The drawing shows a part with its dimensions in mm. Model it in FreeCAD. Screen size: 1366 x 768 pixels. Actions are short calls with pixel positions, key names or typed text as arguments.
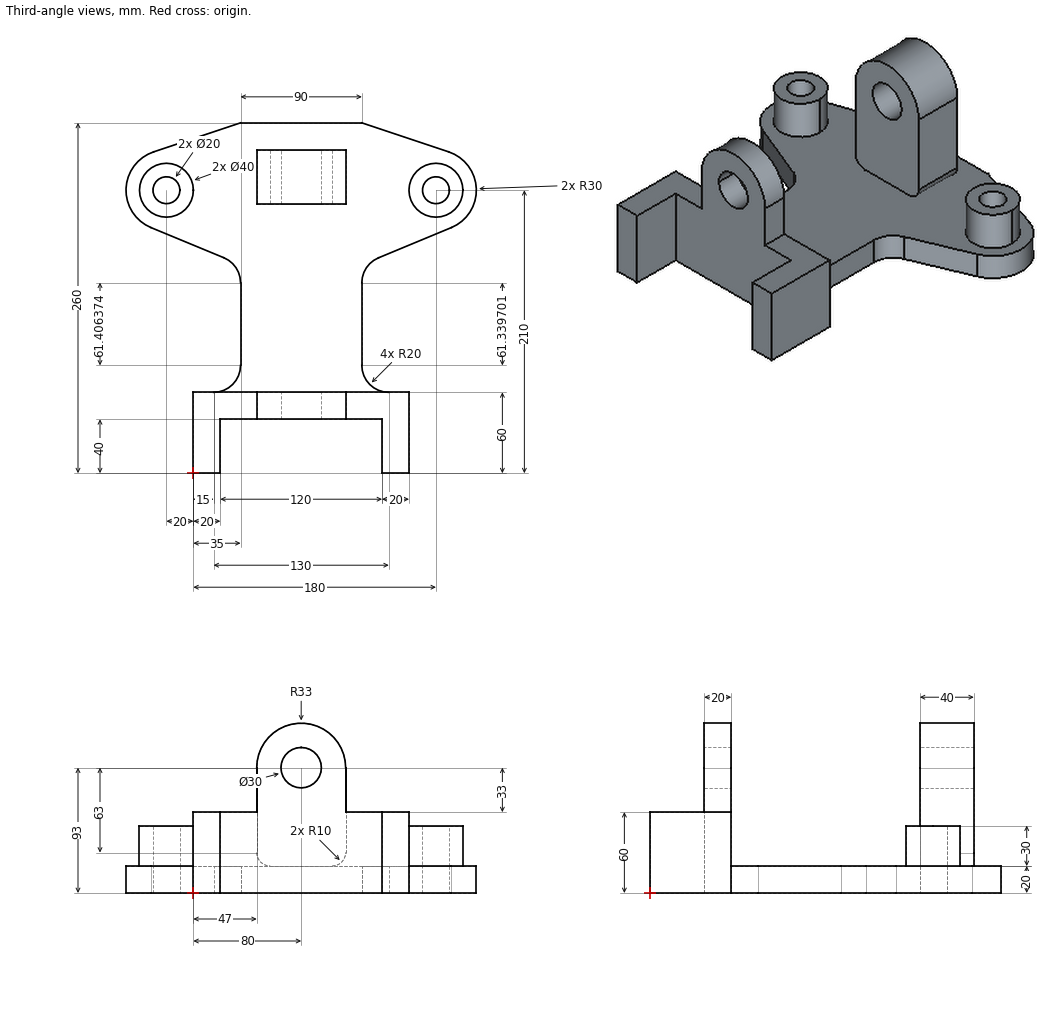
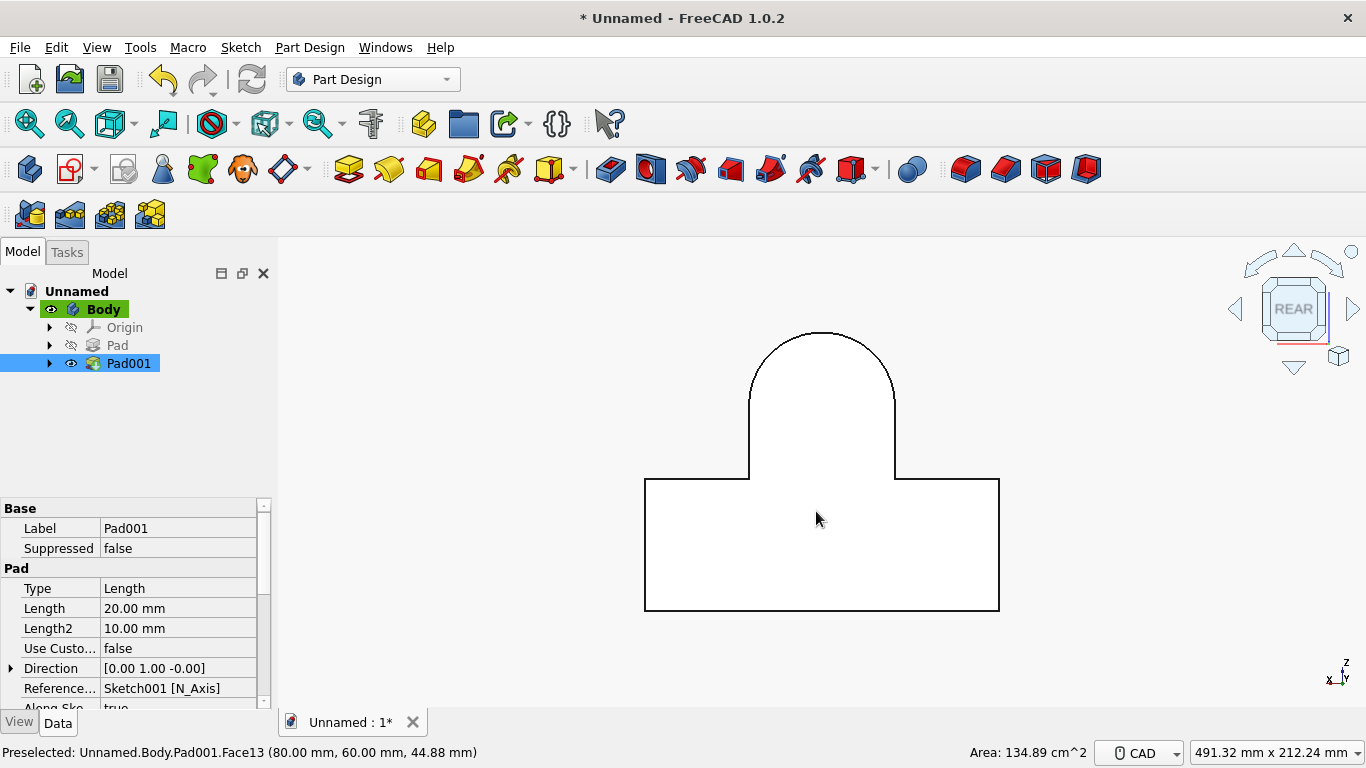
click(70, 170)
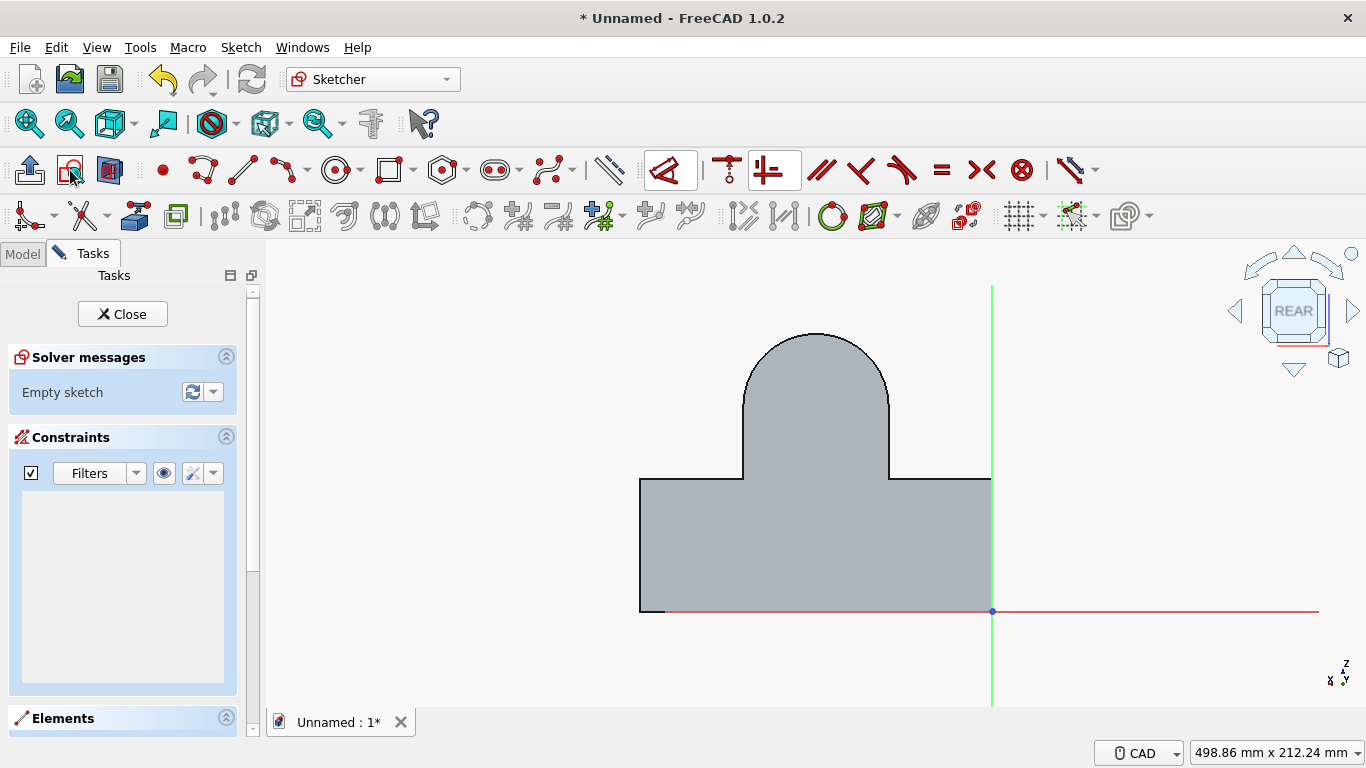
scroll(838, 385, up, 7)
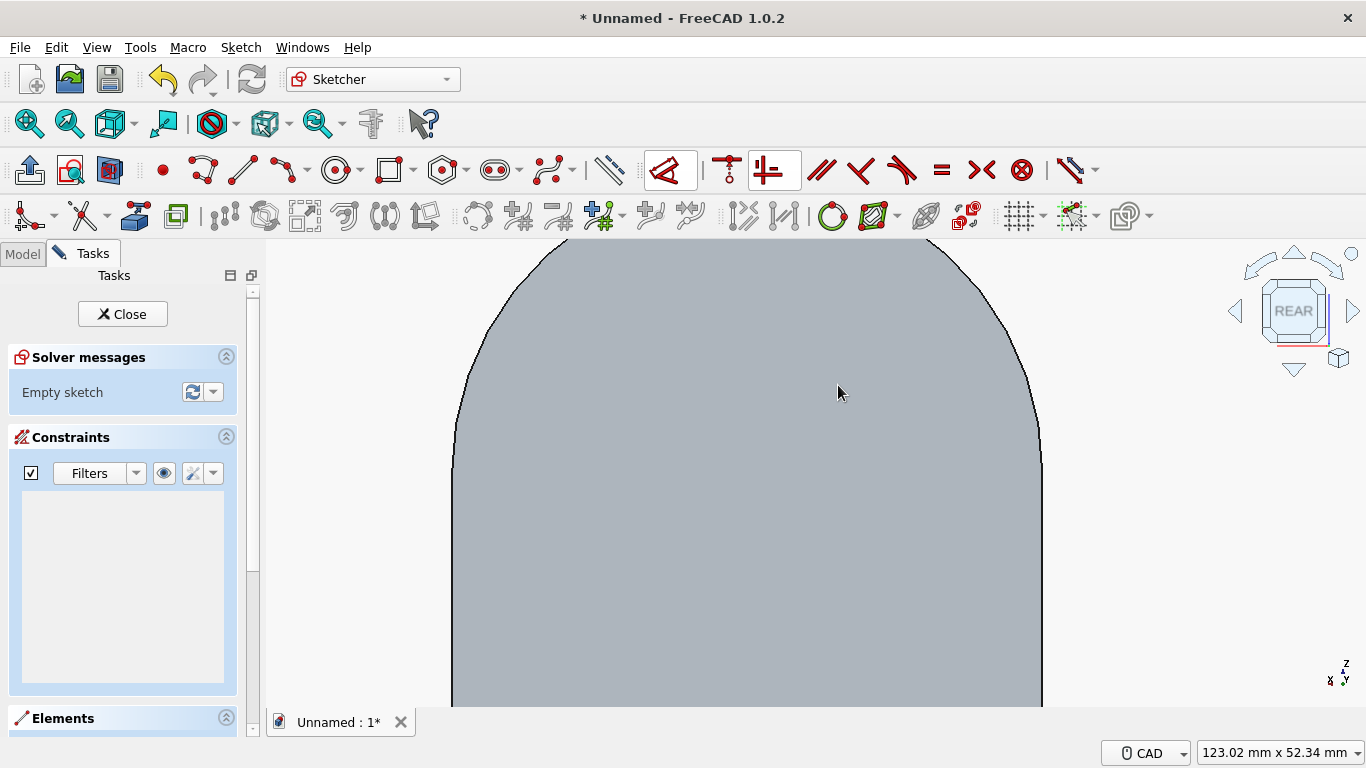
click(336, 170)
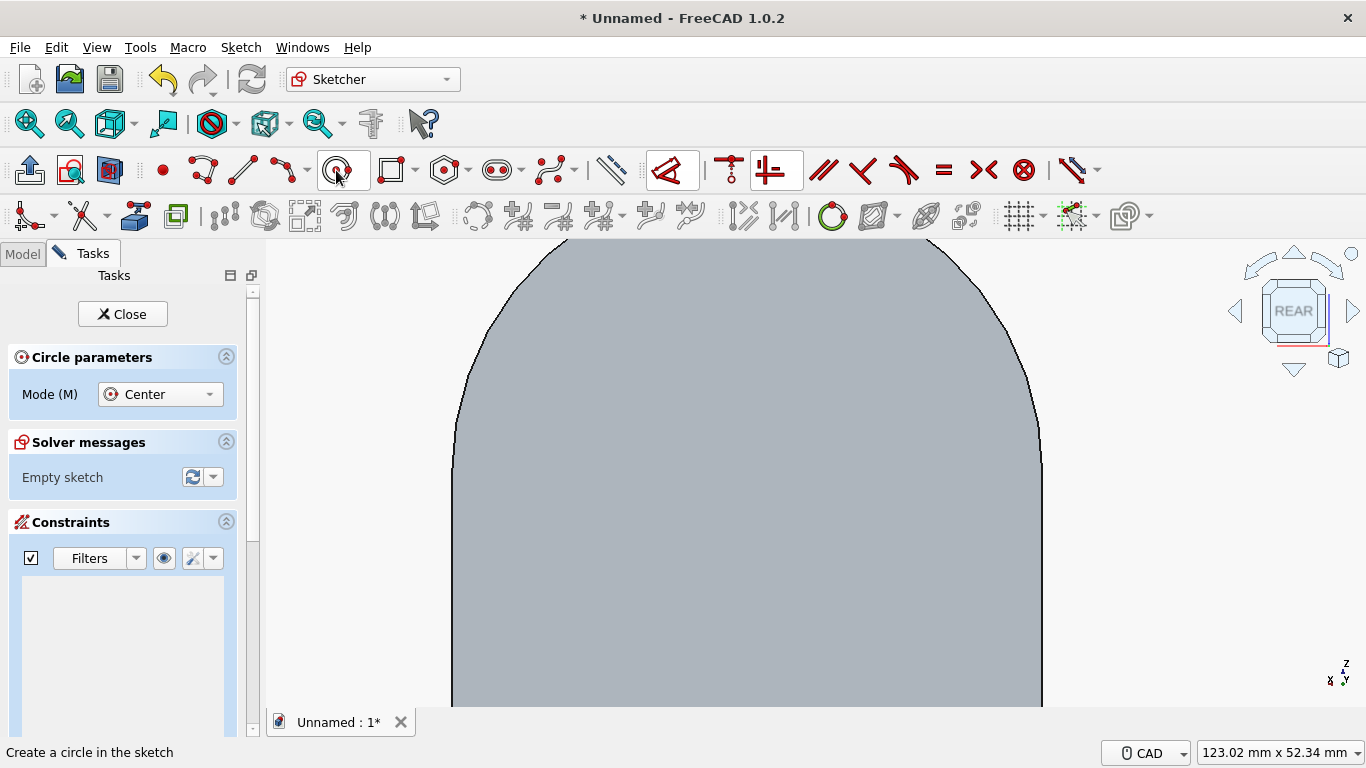
click(747, 472)
click(842, 377)
key(Escape)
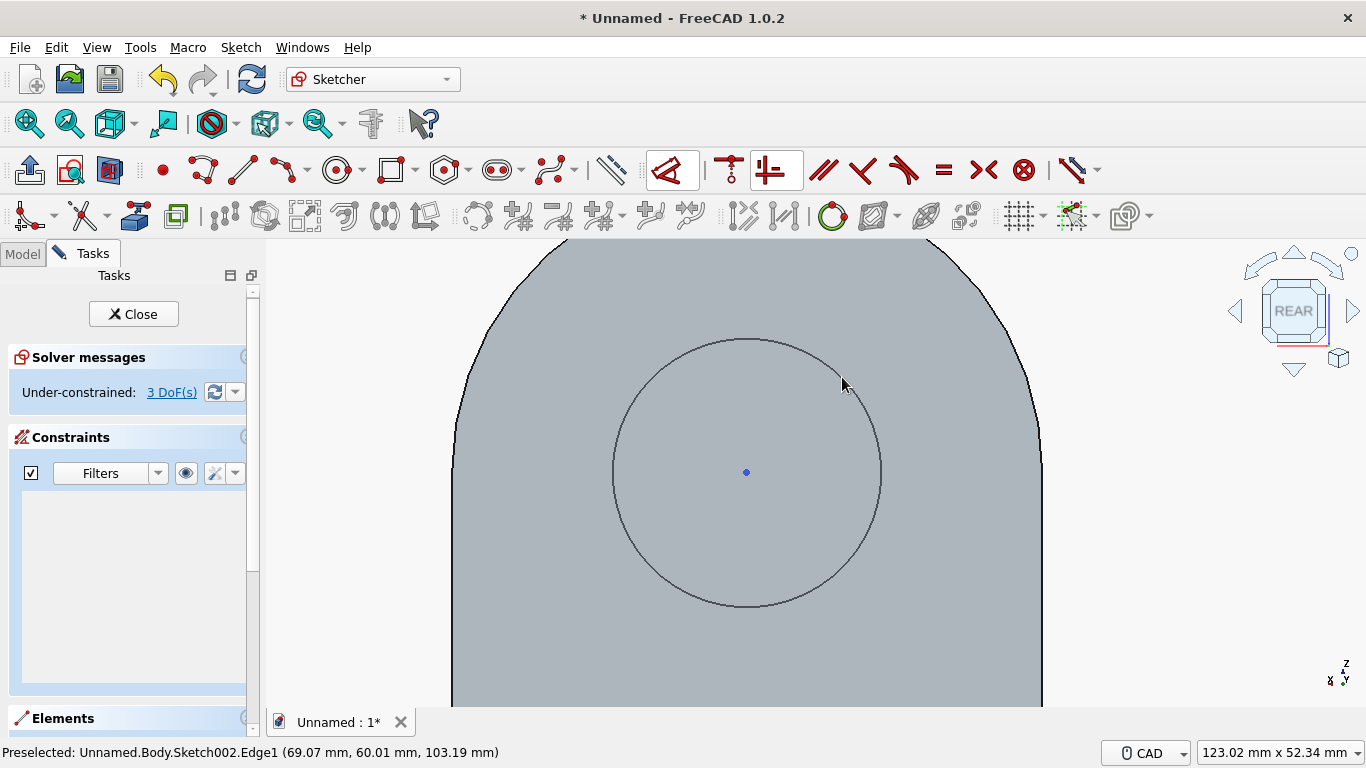
click(842, 378)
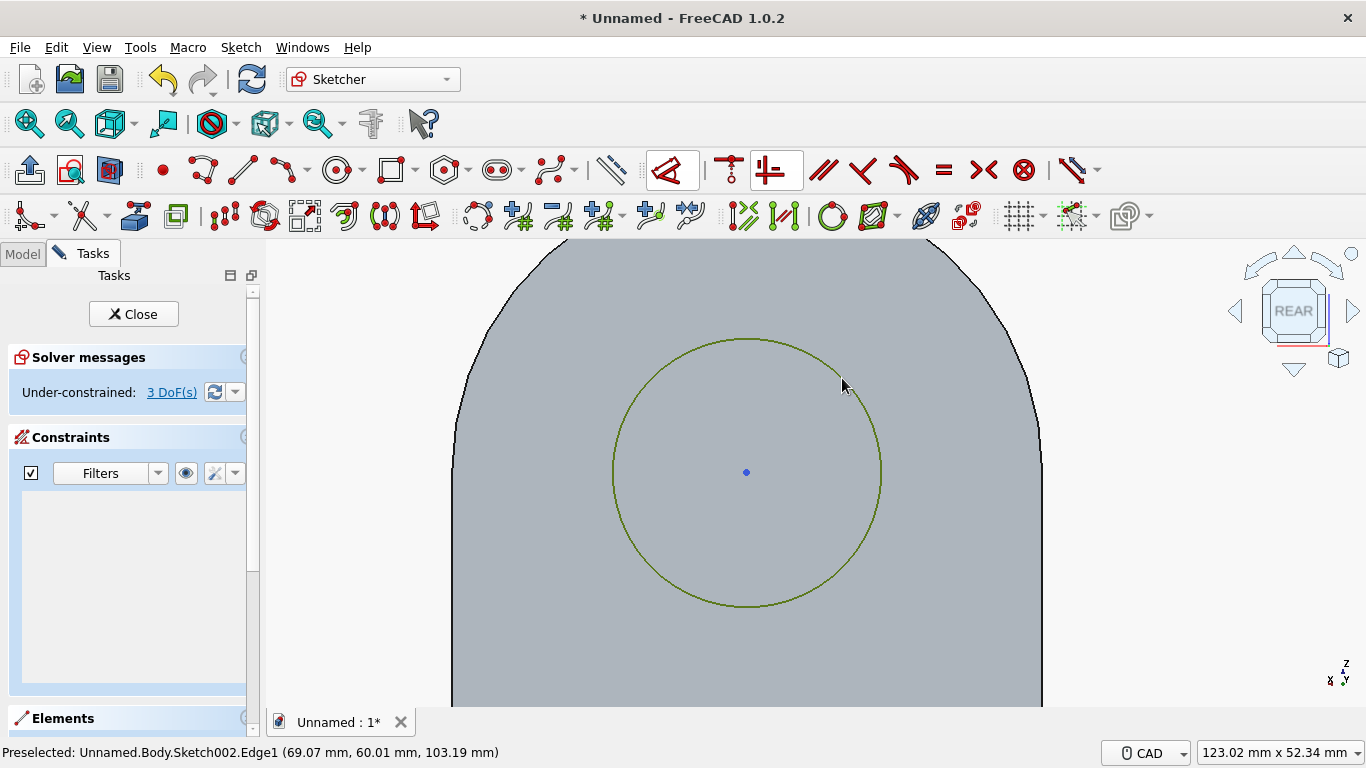
click(694, 170)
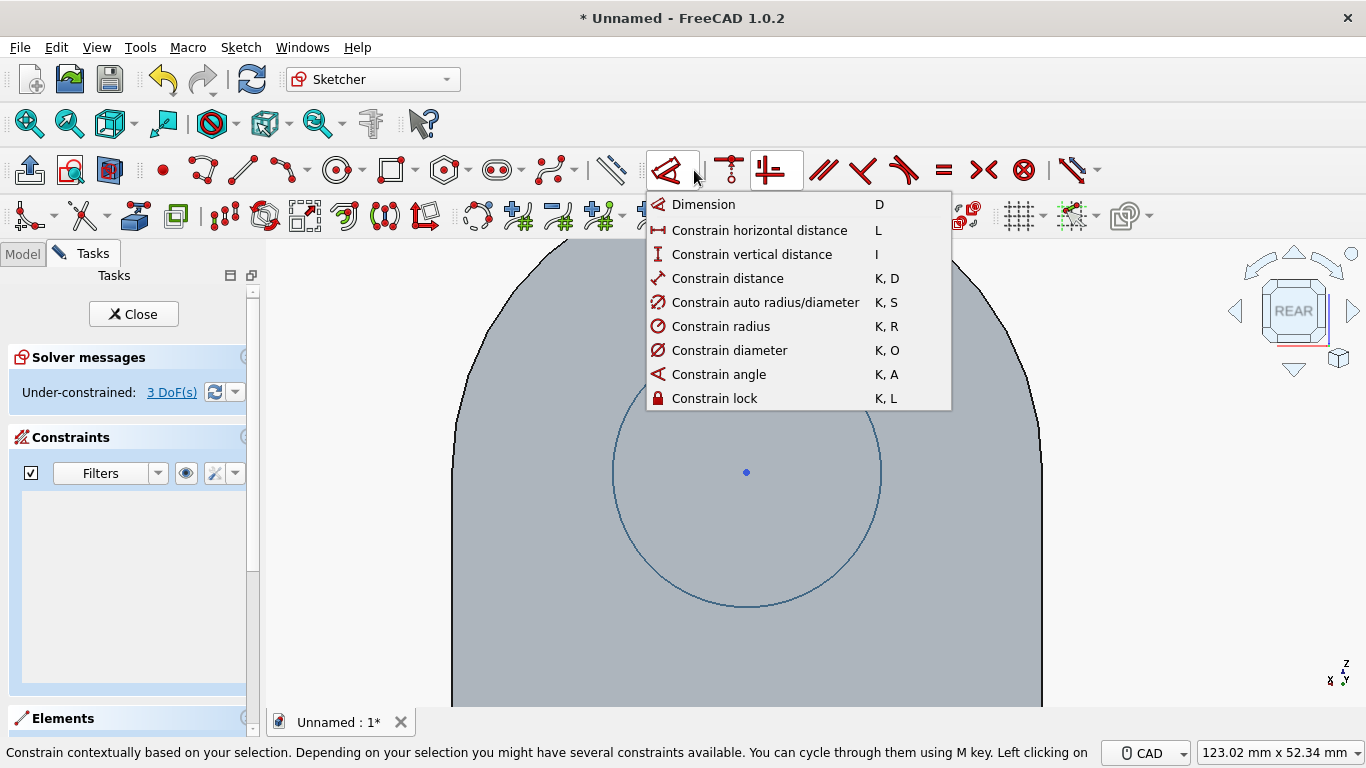
click(799, 350)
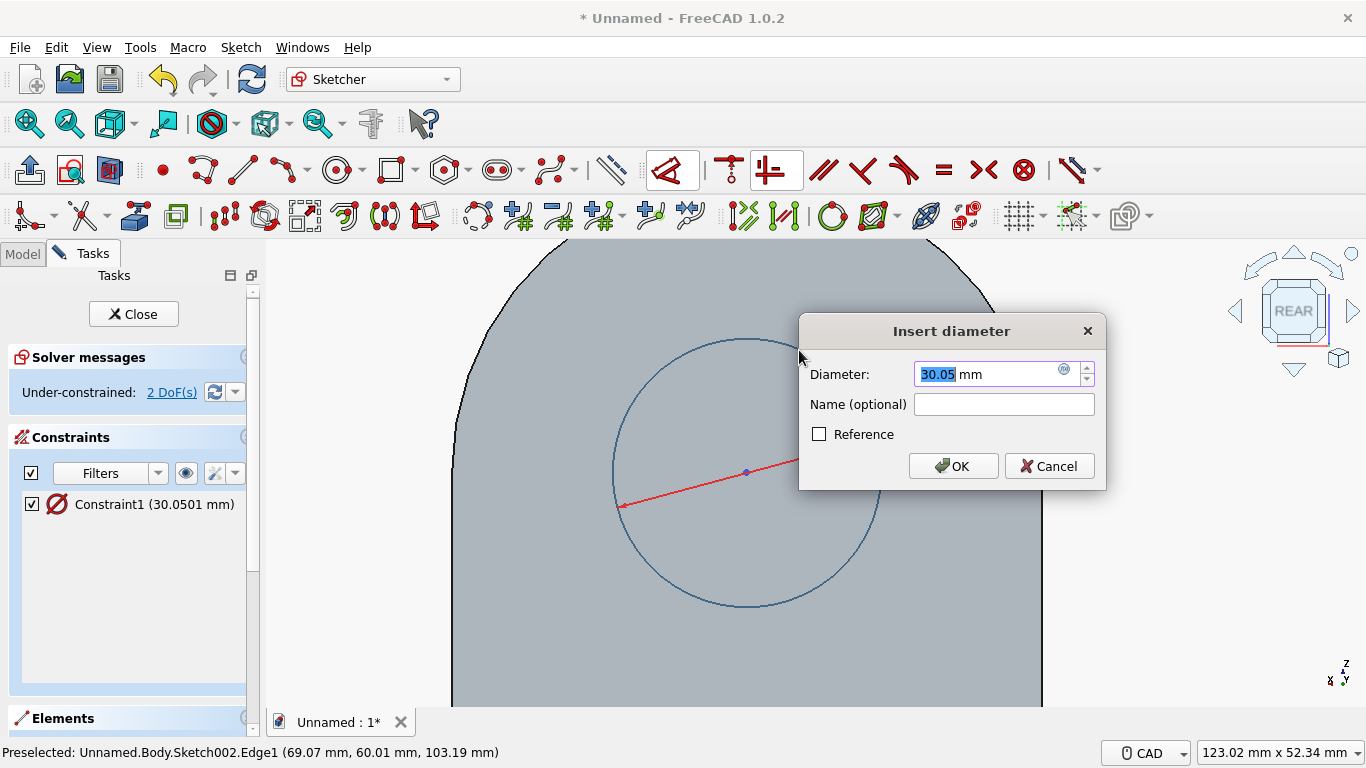
text(30)
key(Return)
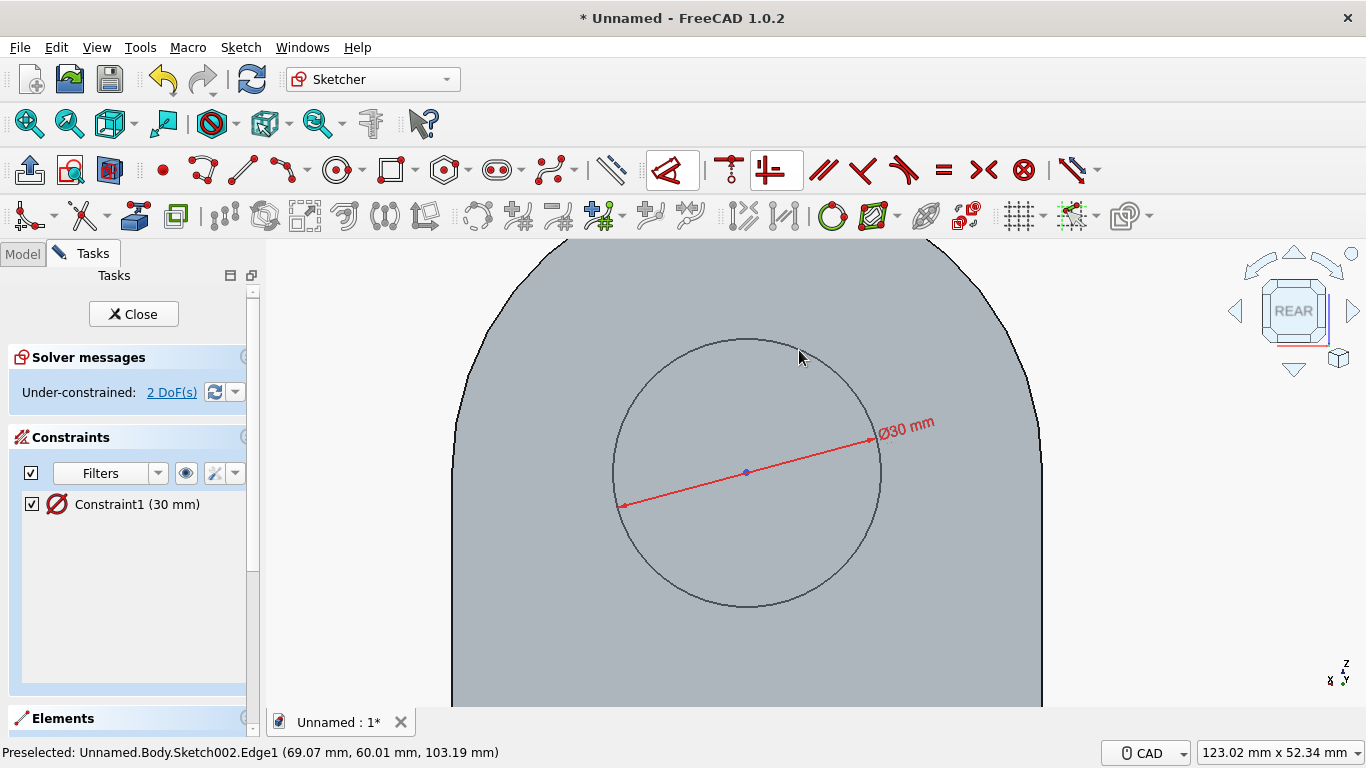
click(747, 473)